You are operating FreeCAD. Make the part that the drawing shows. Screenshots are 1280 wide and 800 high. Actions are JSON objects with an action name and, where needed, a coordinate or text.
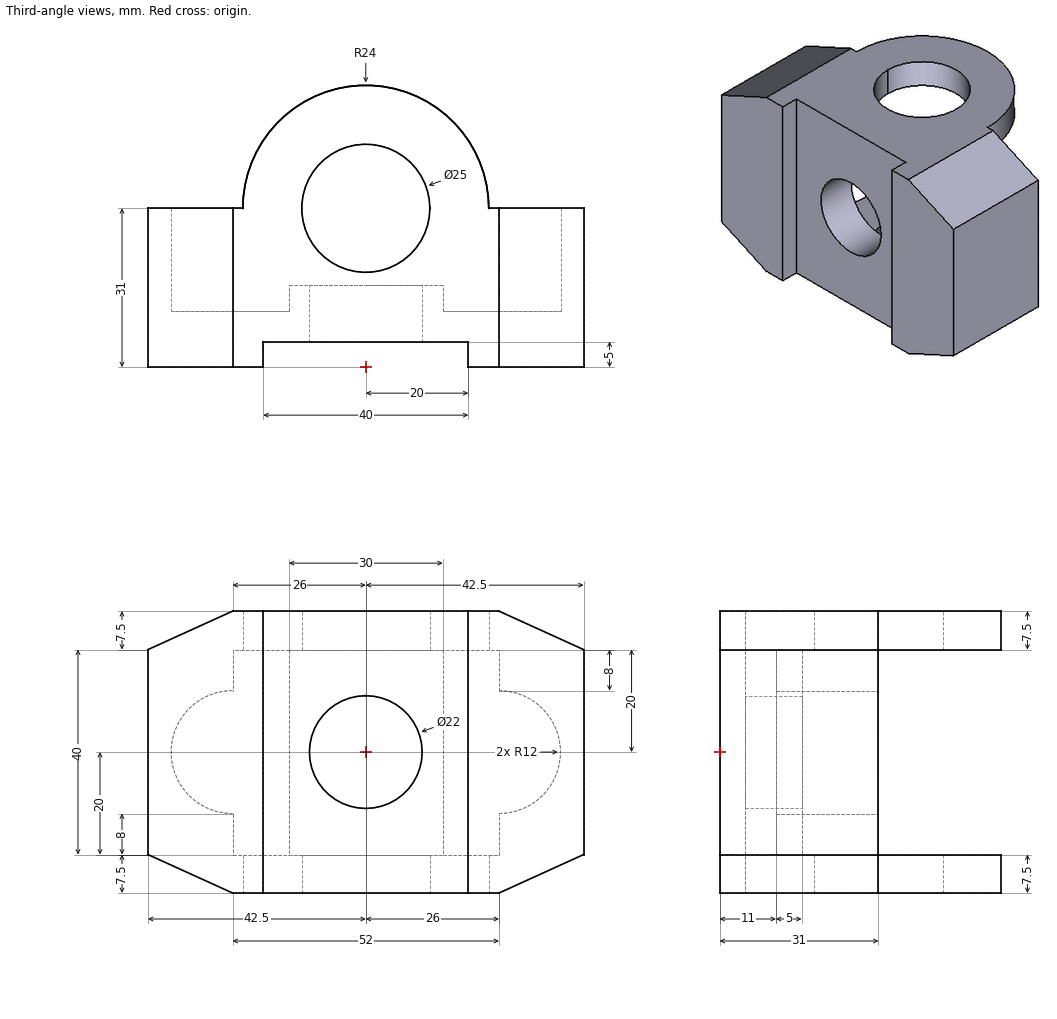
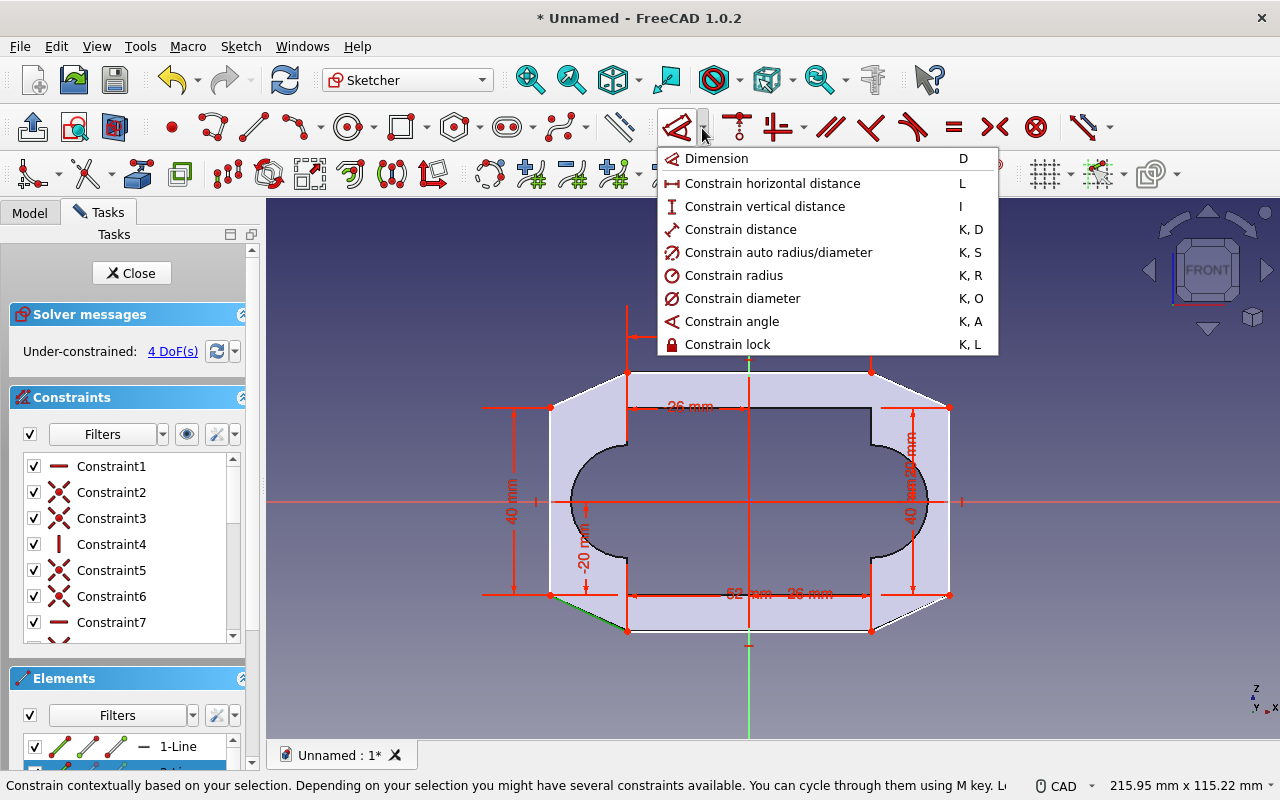
{"action": "left_click", "coordinate": [828, 206]}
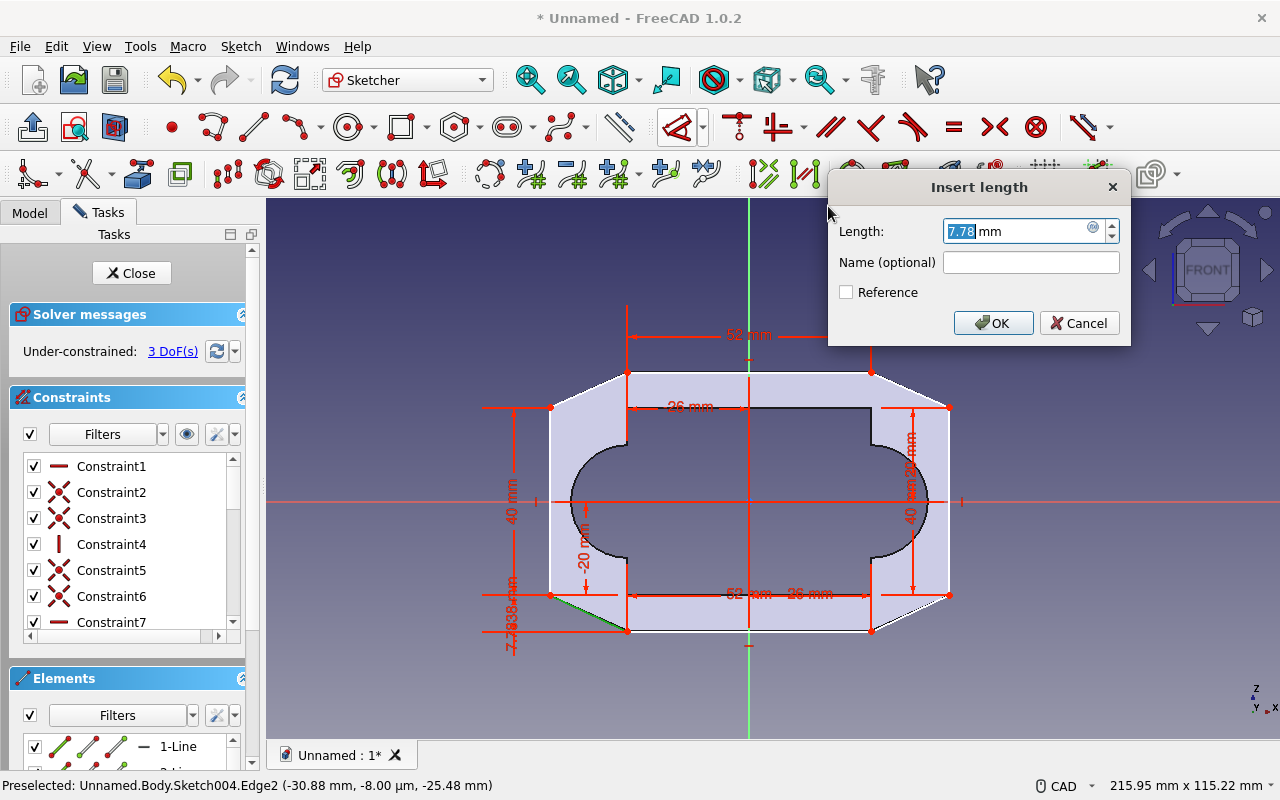
{"action": "type", "text": "7.5"}
{"action": "key", "text": "Return"}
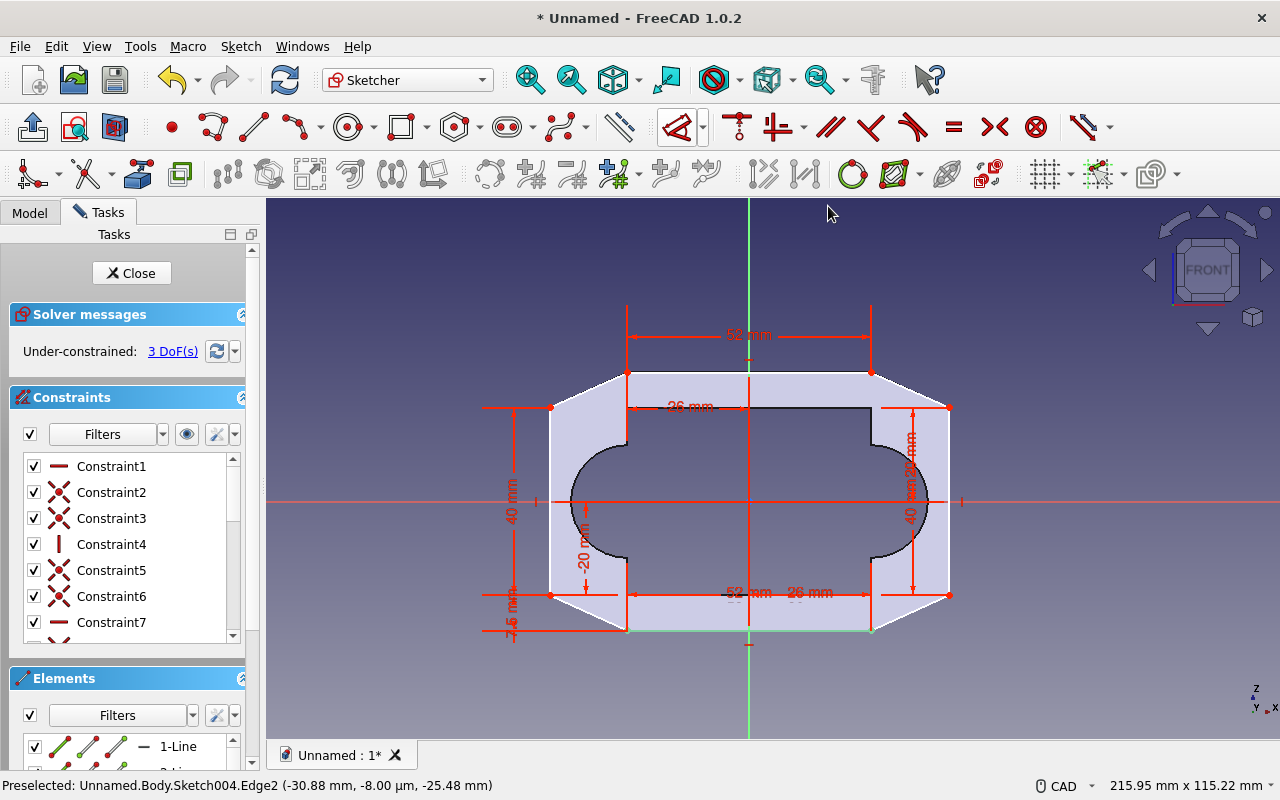
{"action": "left_click", "coordinate": [573, 397]}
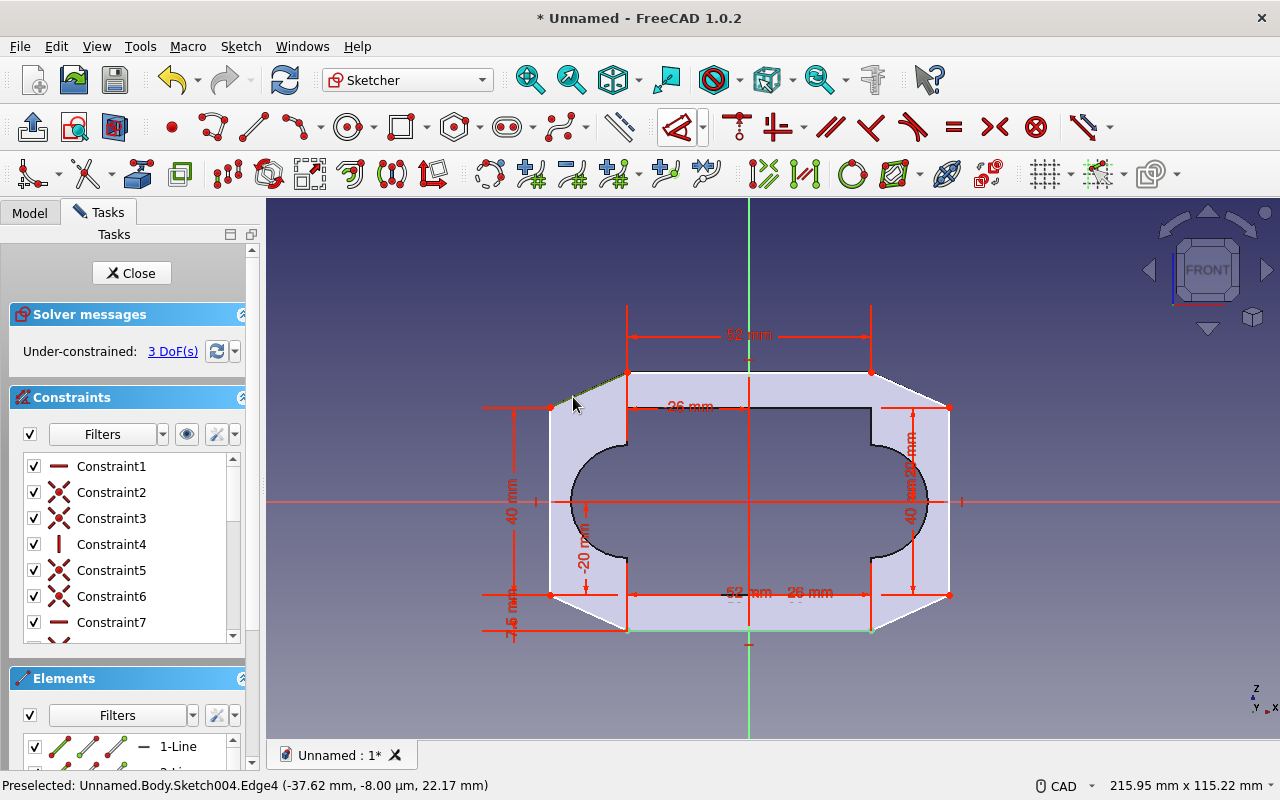
{"action": "key", "text": "i"}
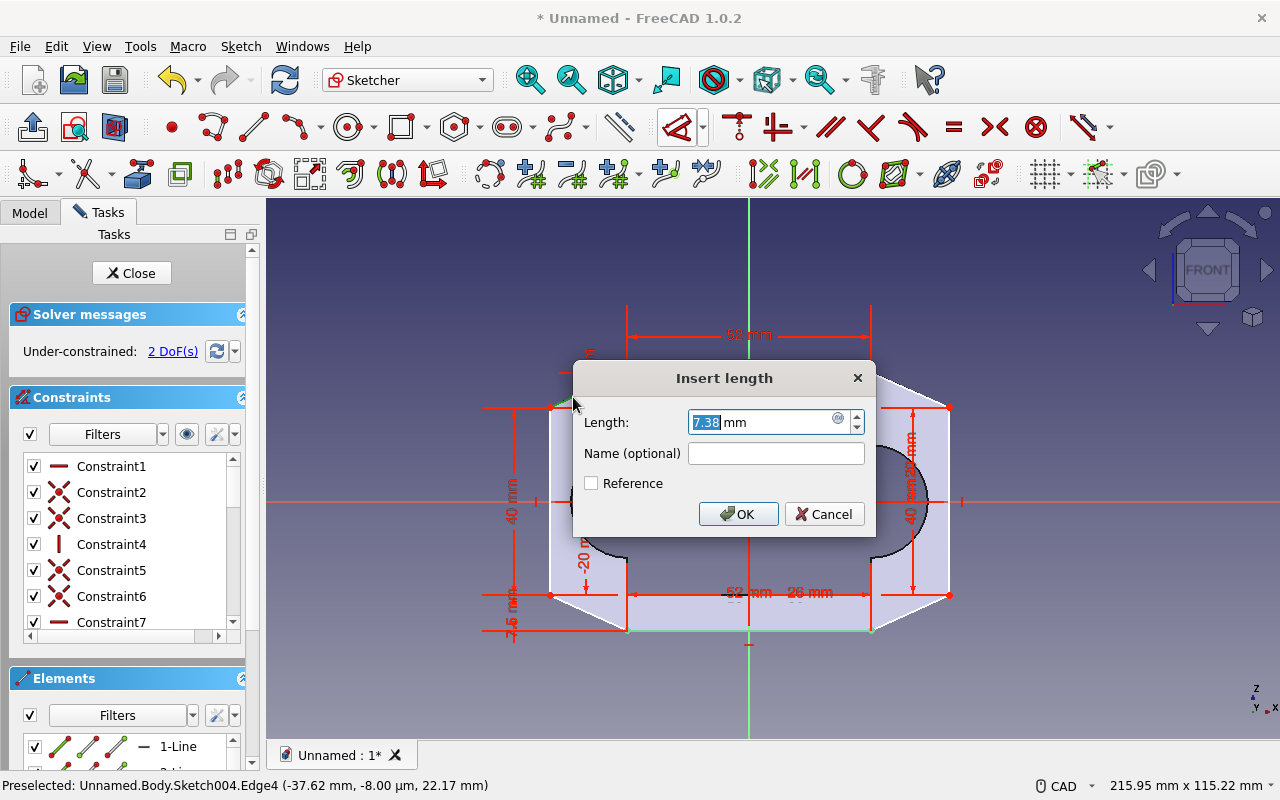
{"action": "type", "text": "7.5"}
{"action": "key", "text": "Return"}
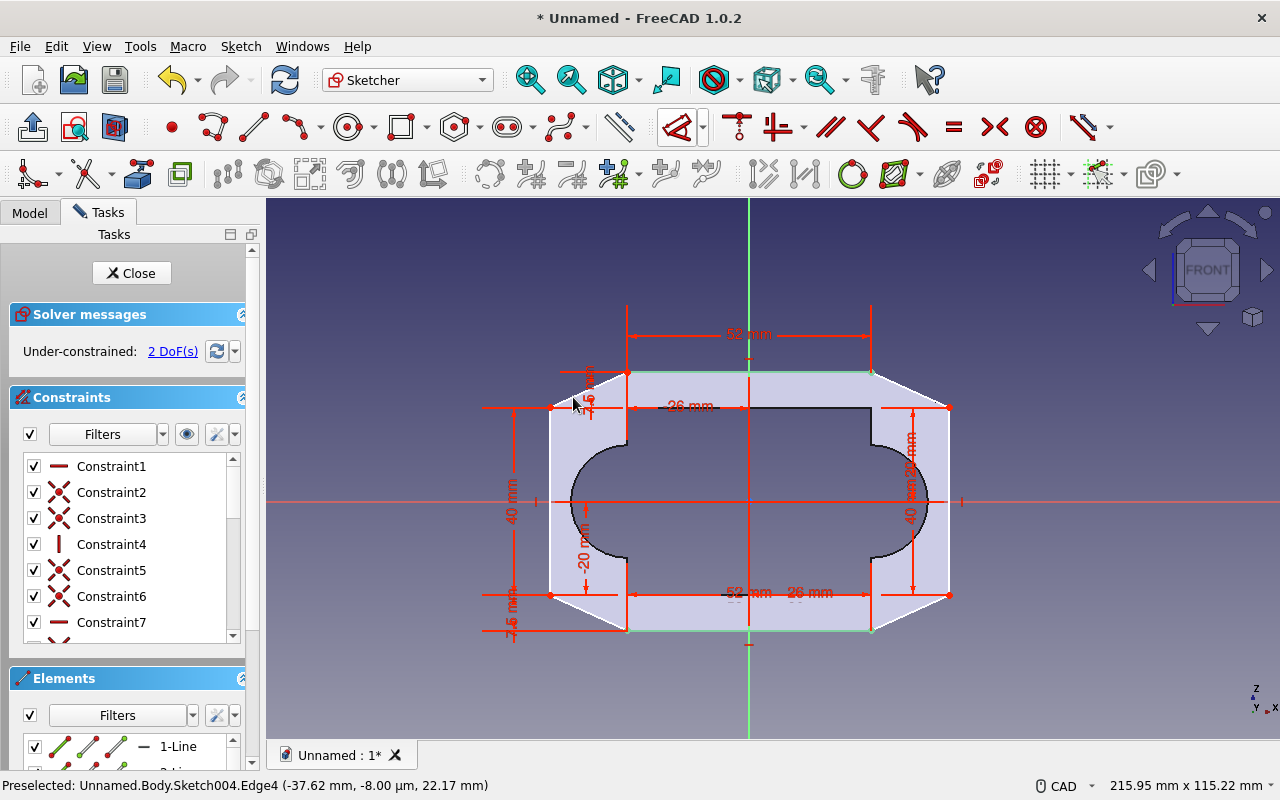
{"action": "left_click", "coordinate": [550, 595]}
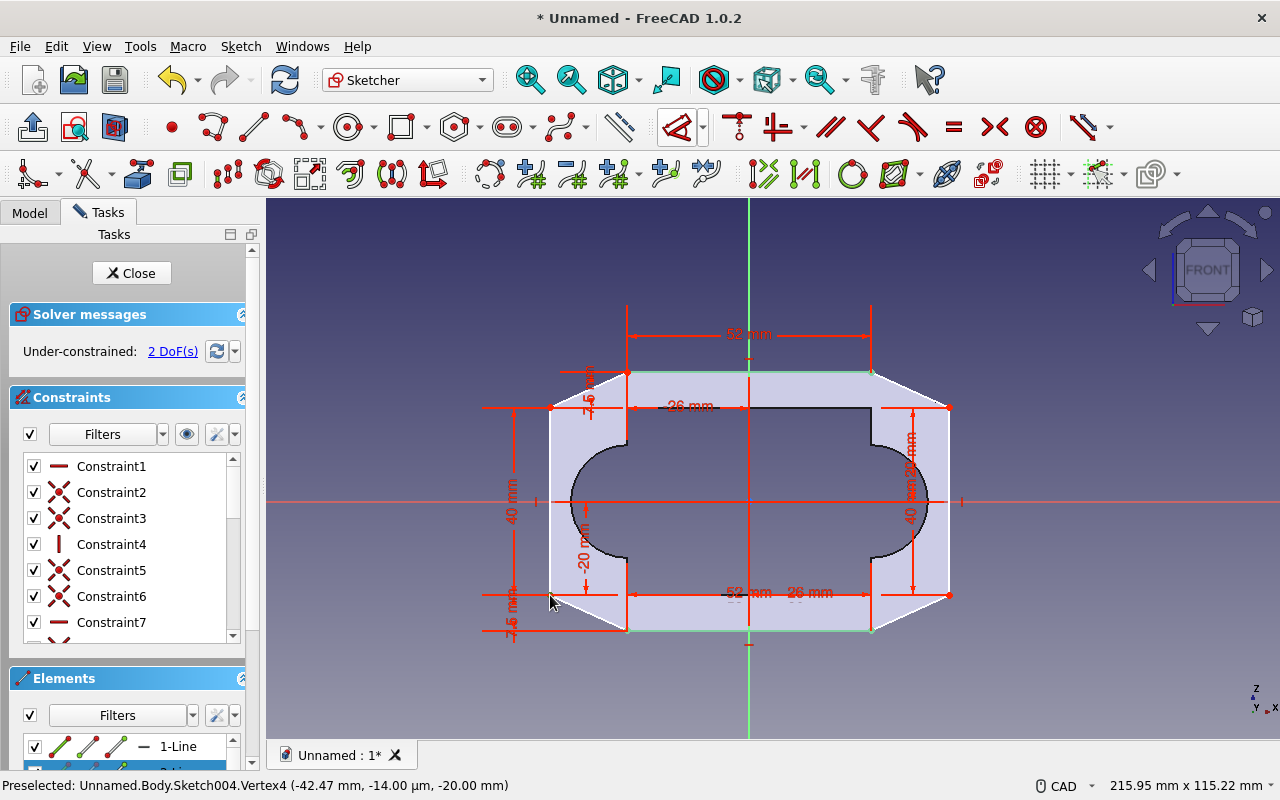
{"action": "key", "text": "l"}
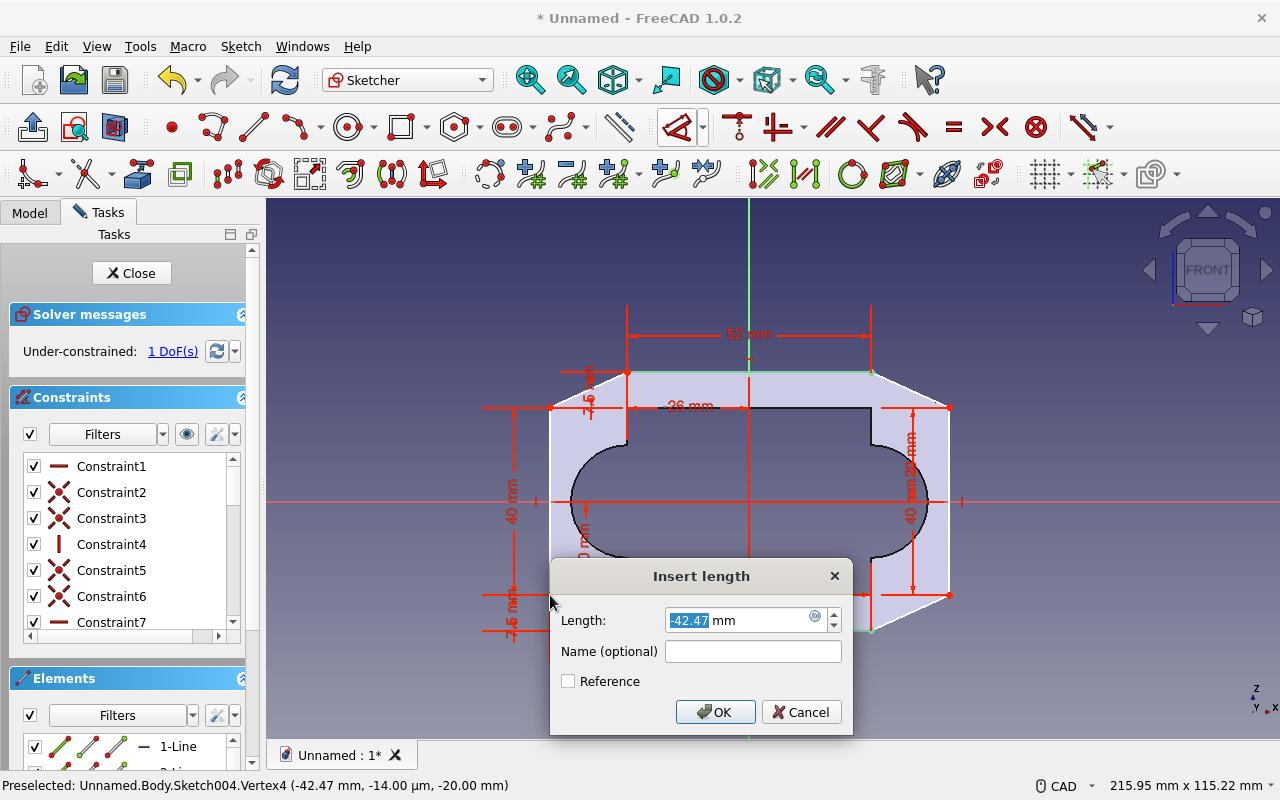
{"action": "type", "text": "-42.5"}
{"action": "key", "text": "Return"}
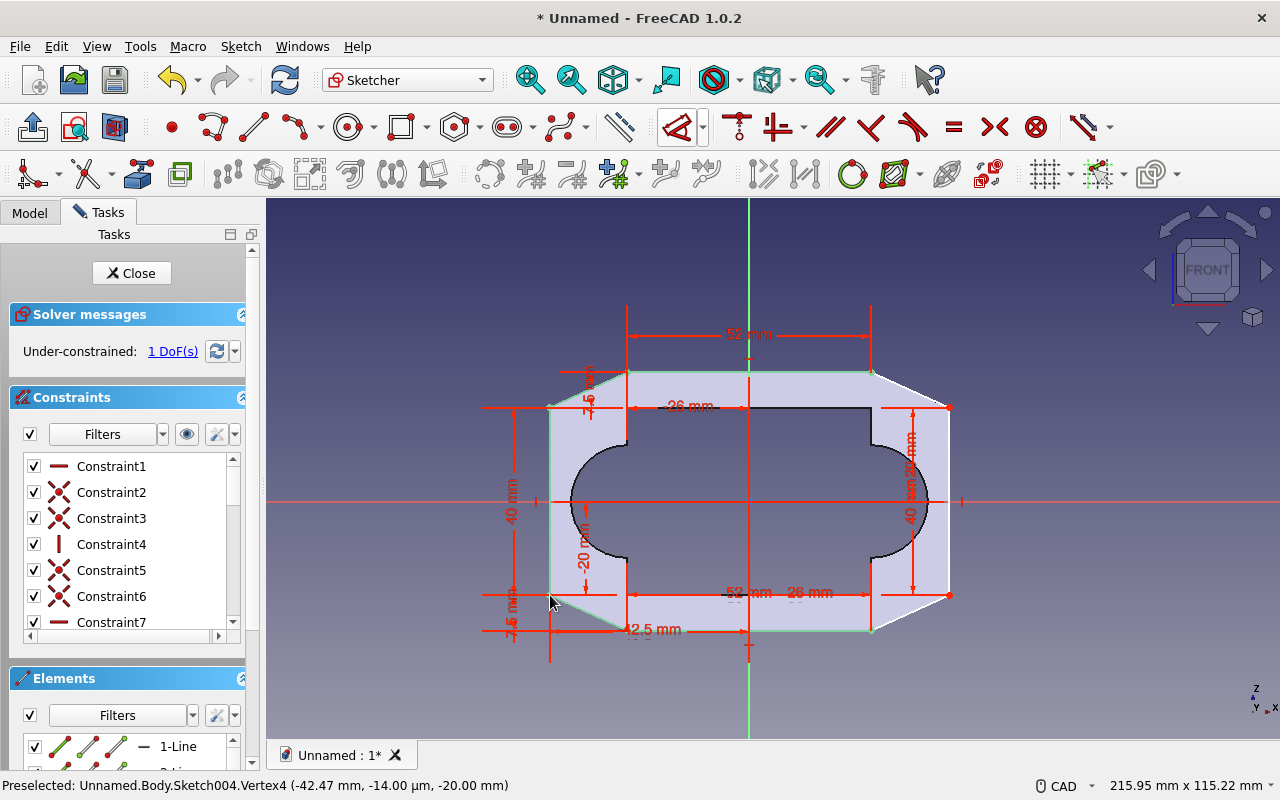
{"action": "left_click", "coordinate": [949, 408]}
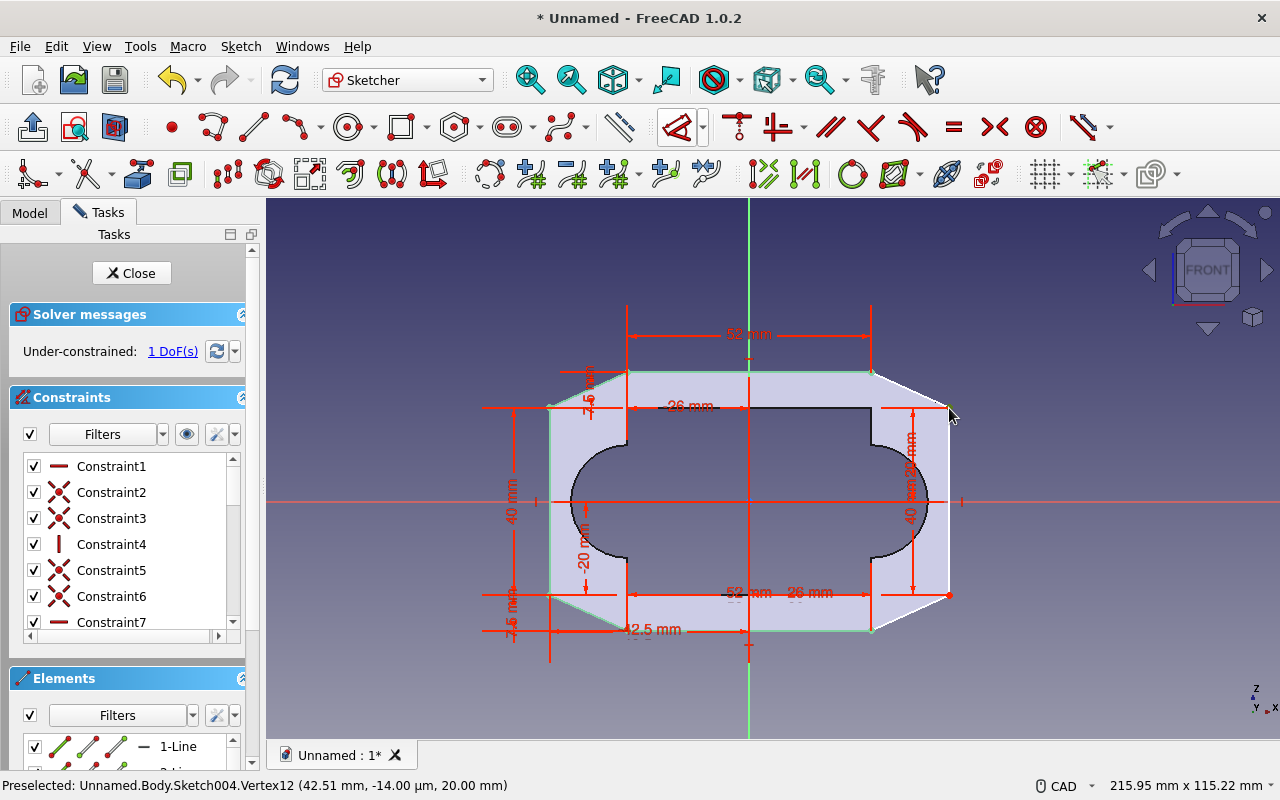
{"action": "left_click", "coordinate": [702, 128]}